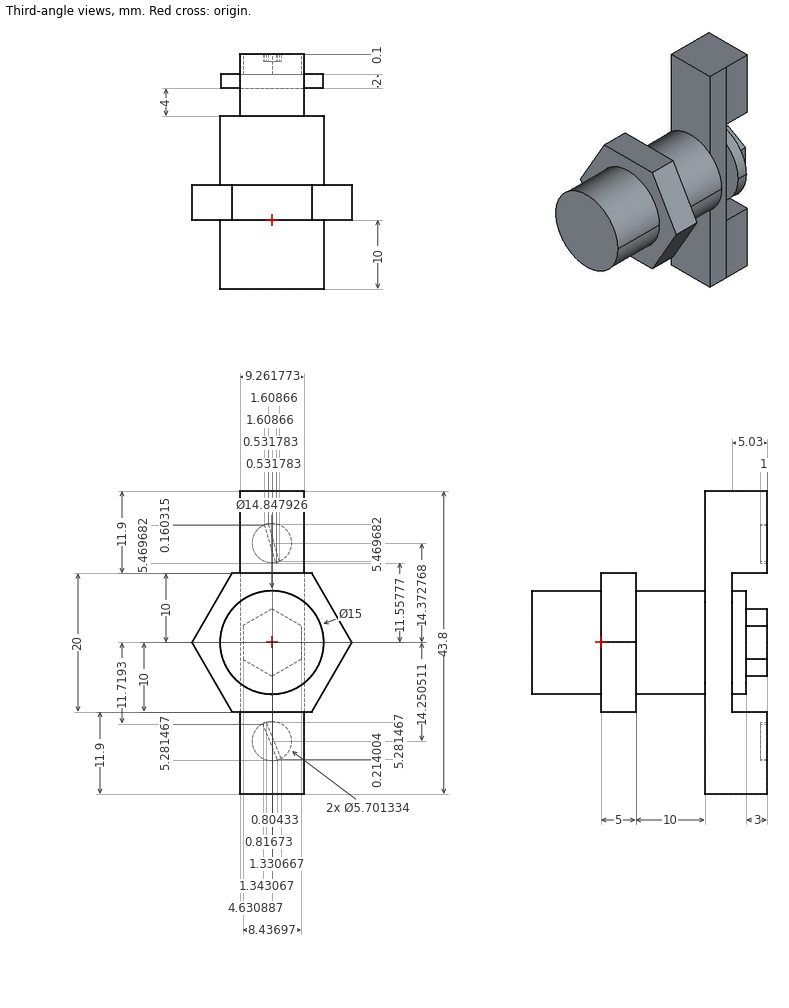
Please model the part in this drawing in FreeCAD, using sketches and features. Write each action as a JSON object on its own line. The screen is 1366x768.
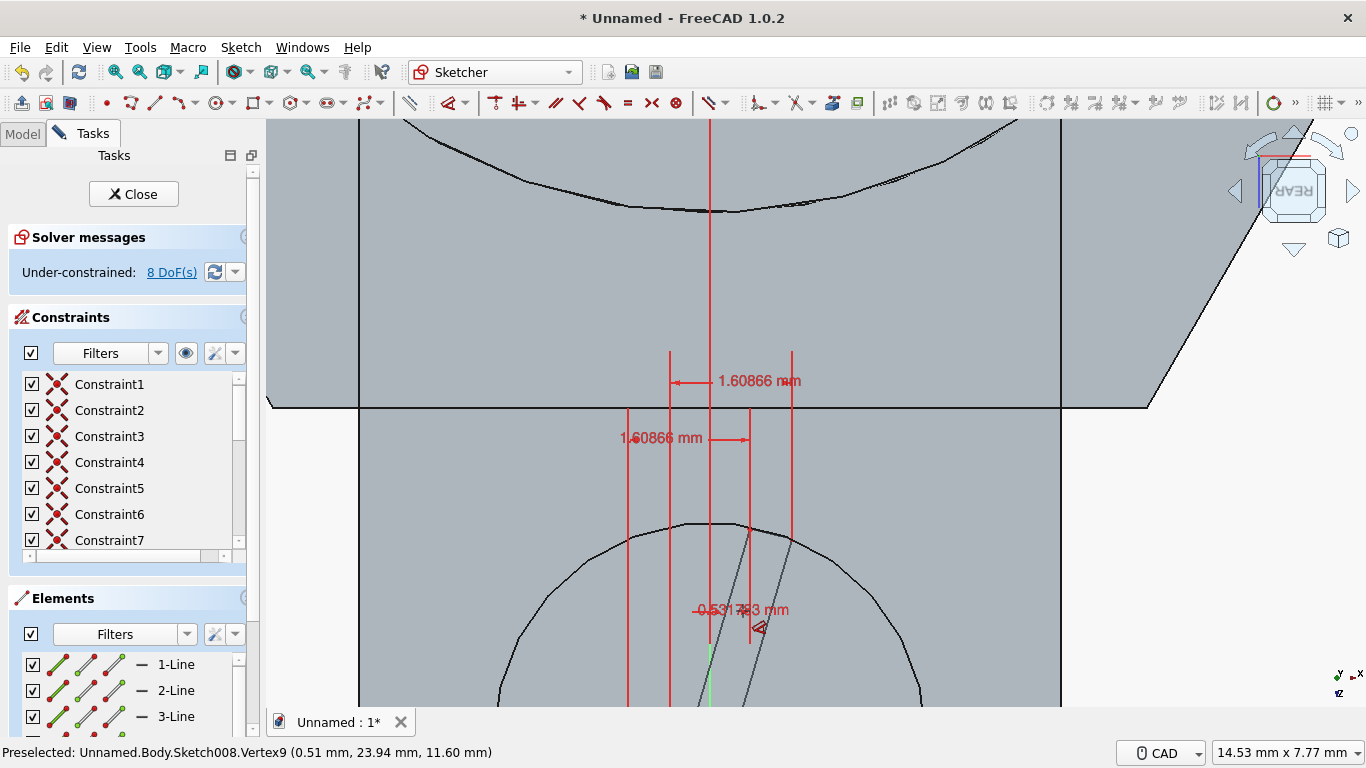
{"action": "scroll", "coordinate": [753, 531], "scroll_direction": "down", "scroll_amount": 10}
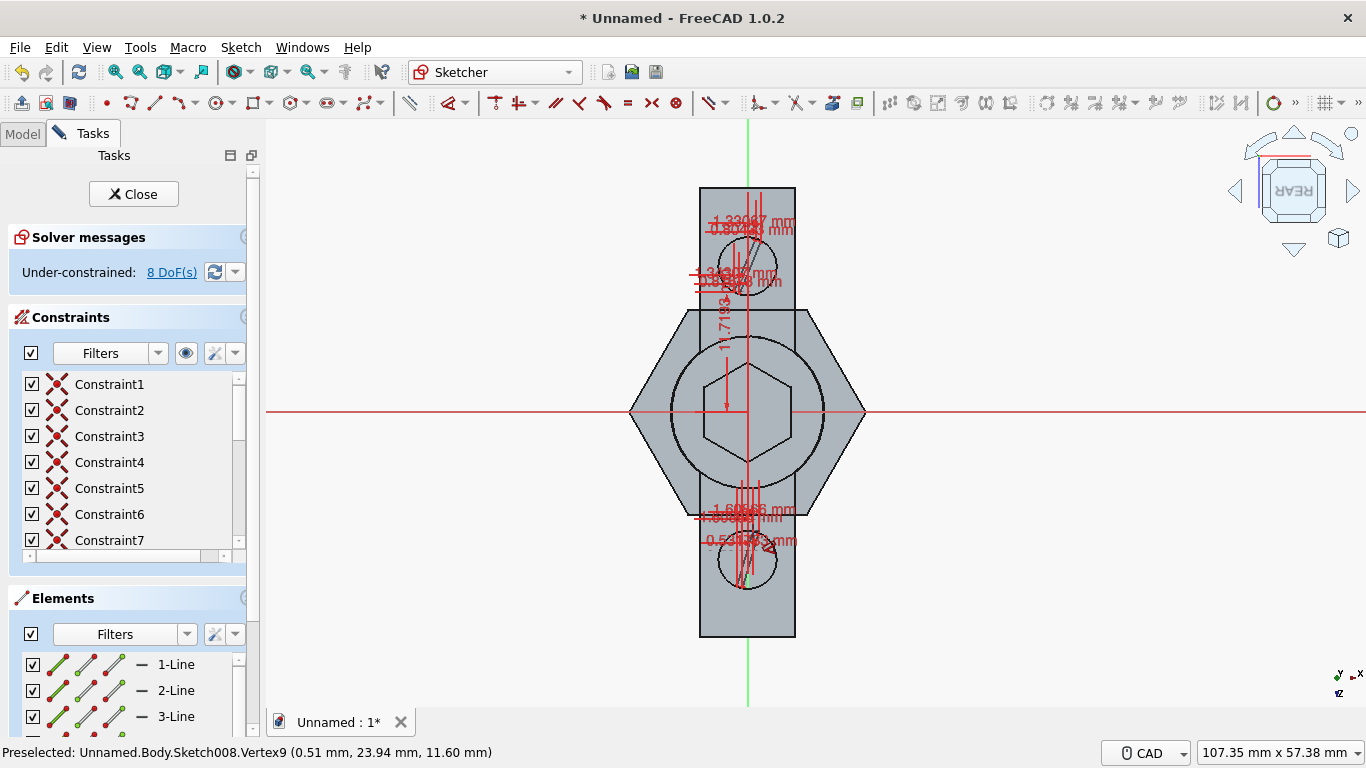
{"action": "scroll", "coordinate": [753, 531], "scroll_direction": "up", "scroll_amount": 4}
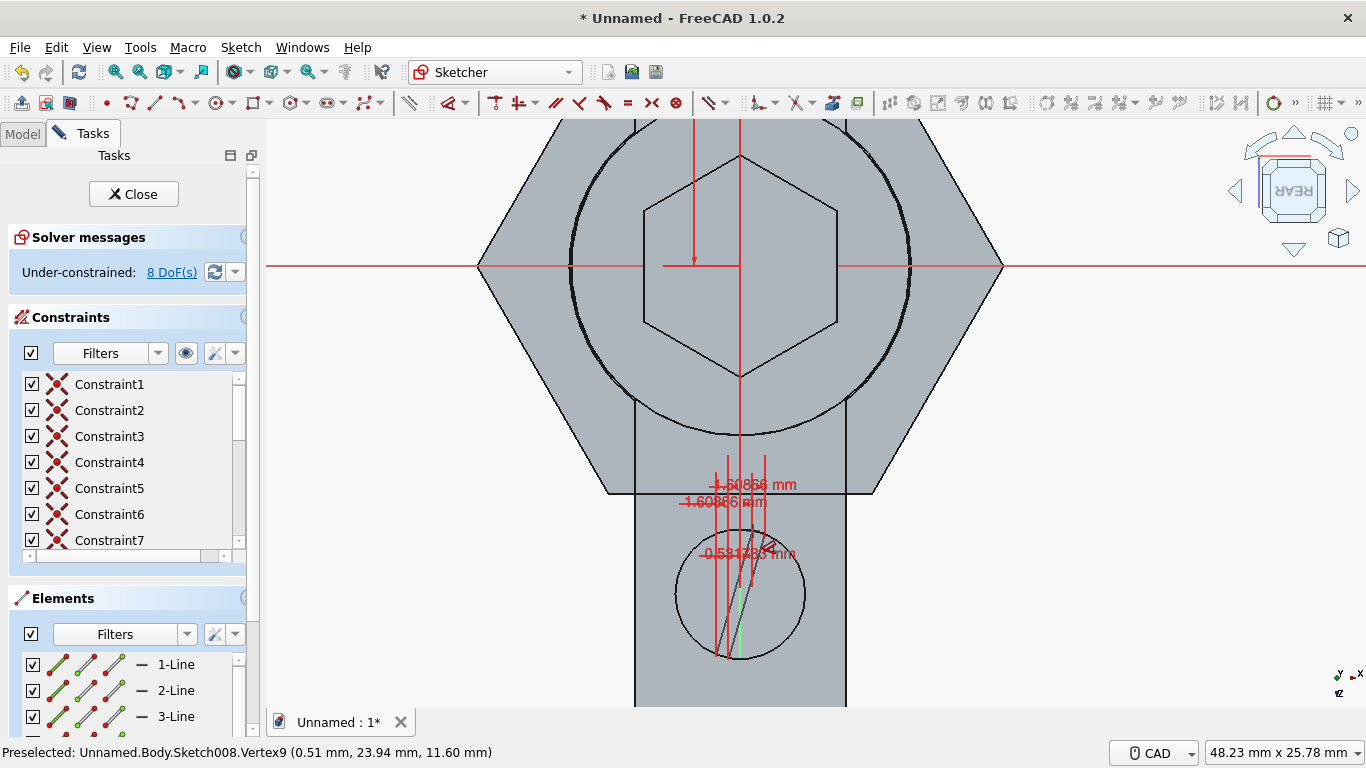
{"action": "left_click", "coordinate": [752, 531]}
{"action": "left_click", "coordinate": [786, 399]}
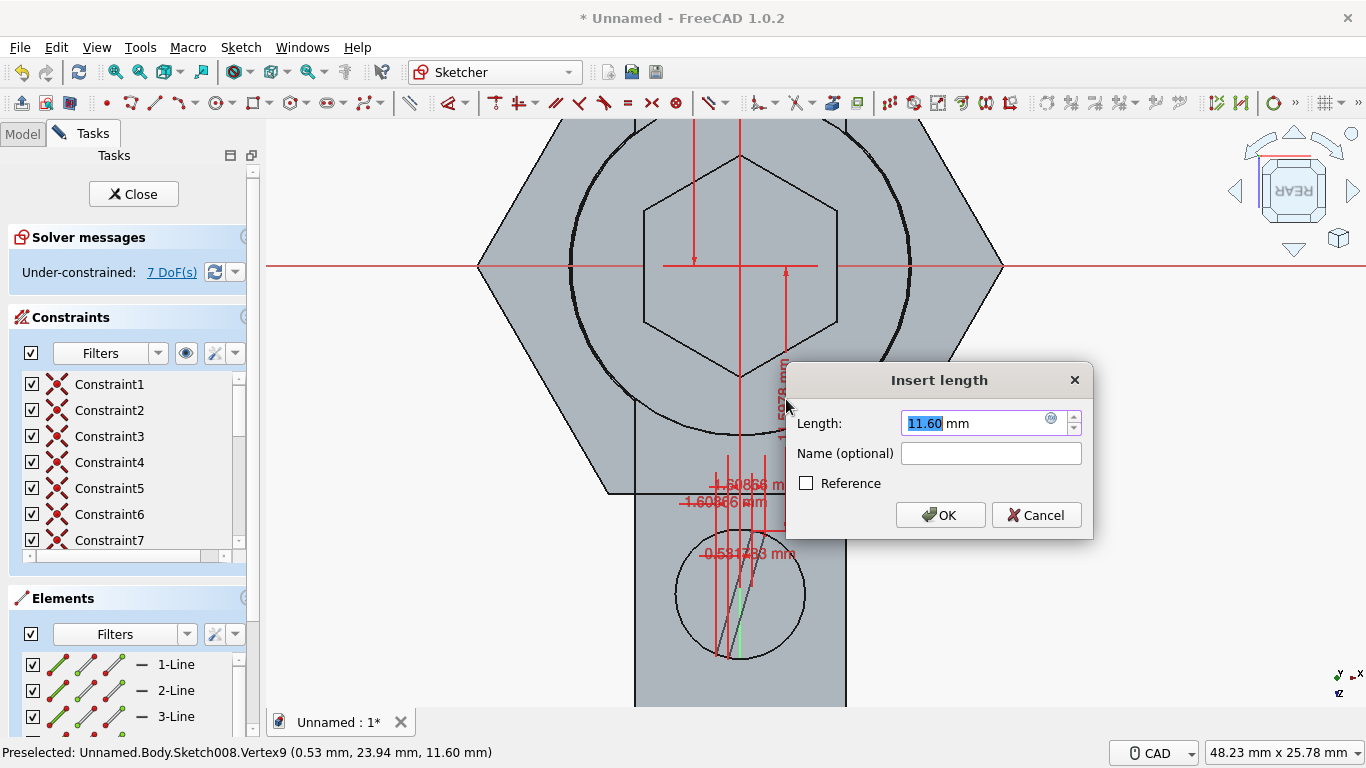
{"action": "type", "text": "11.55777"}
{"action": "key", "text": "Return"}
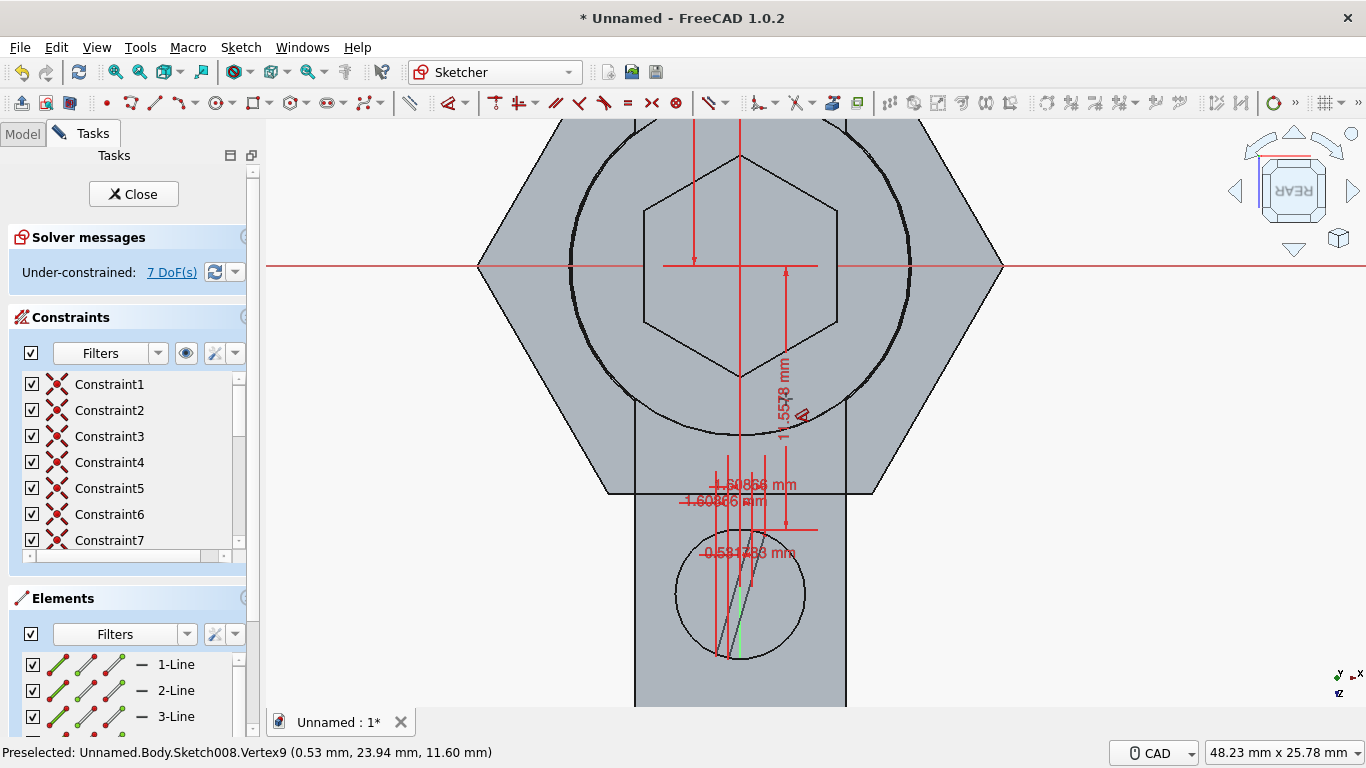
{"action": "scroll", "coordinate": [728, 659], "scroll_direction": "up", "scroll_amount": 6}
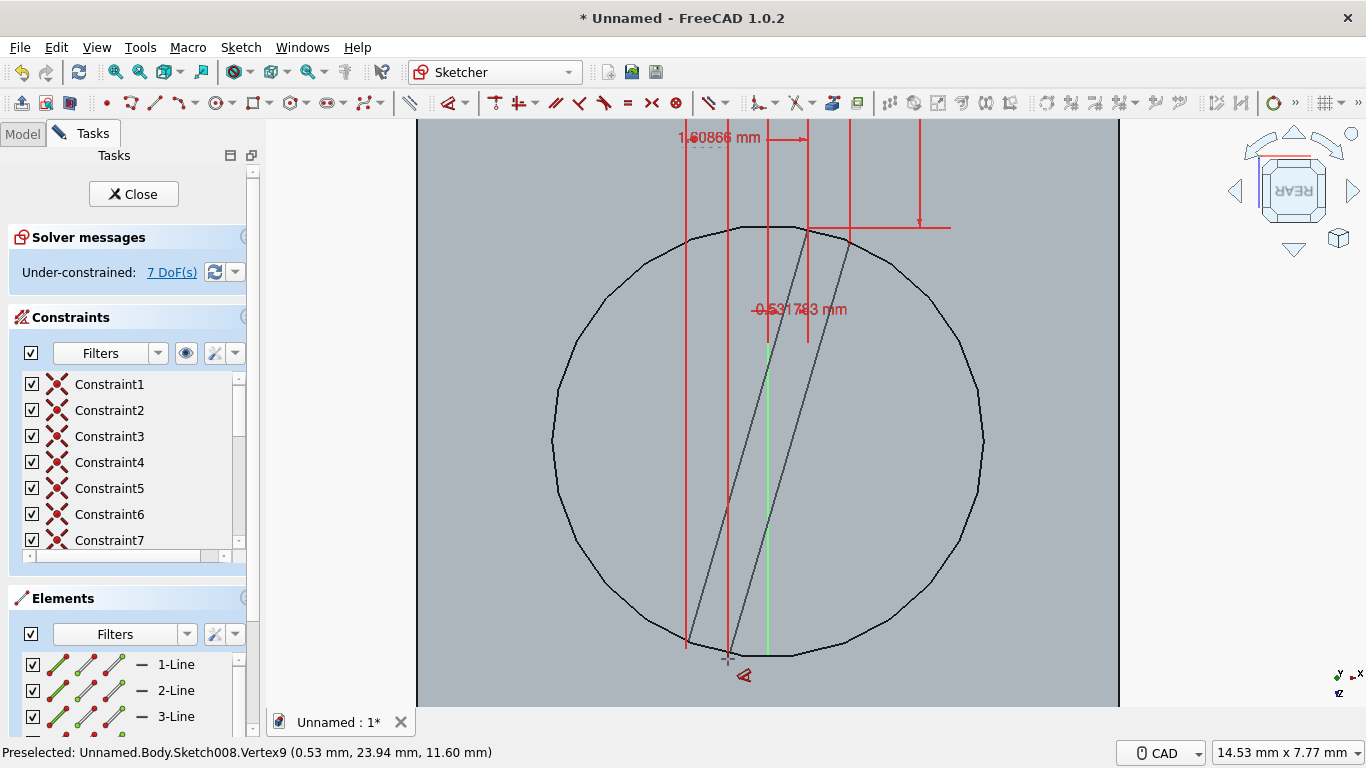
{"action": "left_click", "coordinate": [728, 658]}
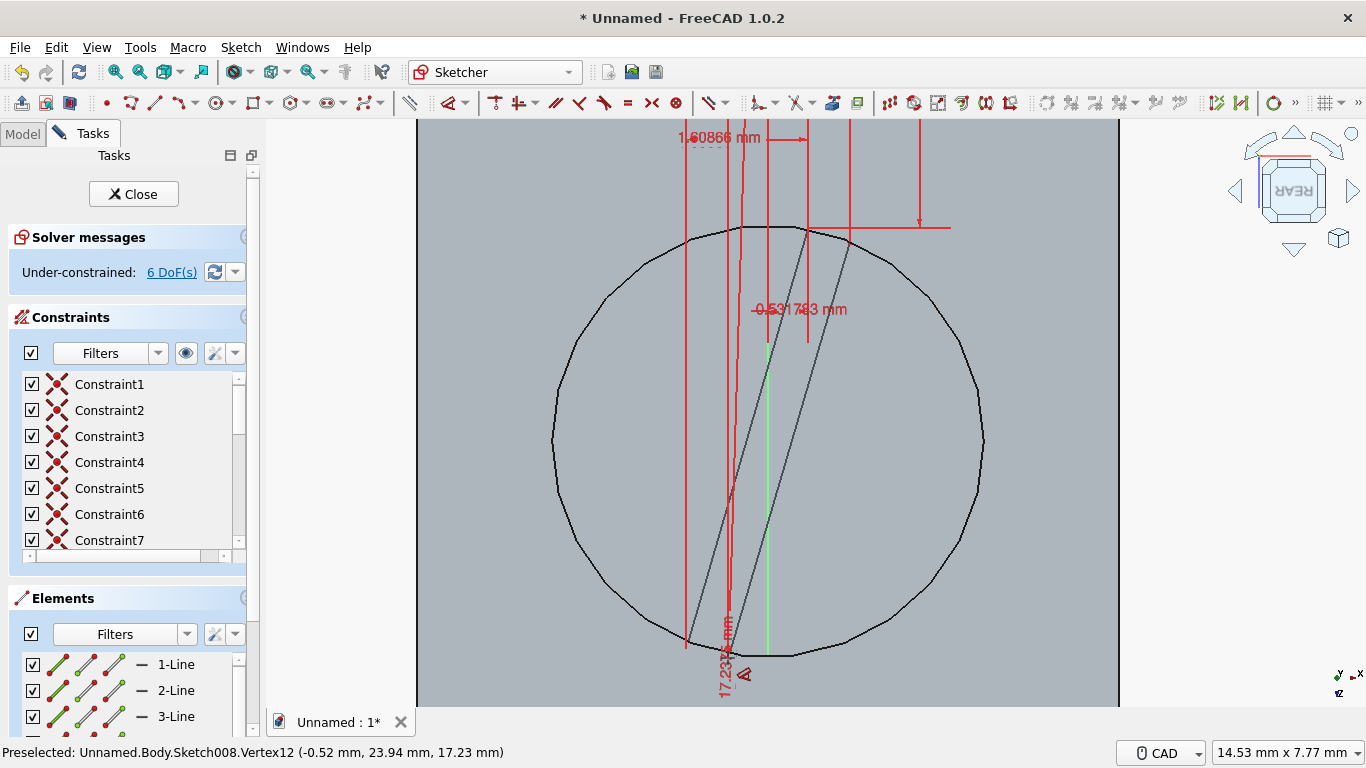
{"action": "key", "text": "Escape"}
{"action": "key", "text": "Escape"}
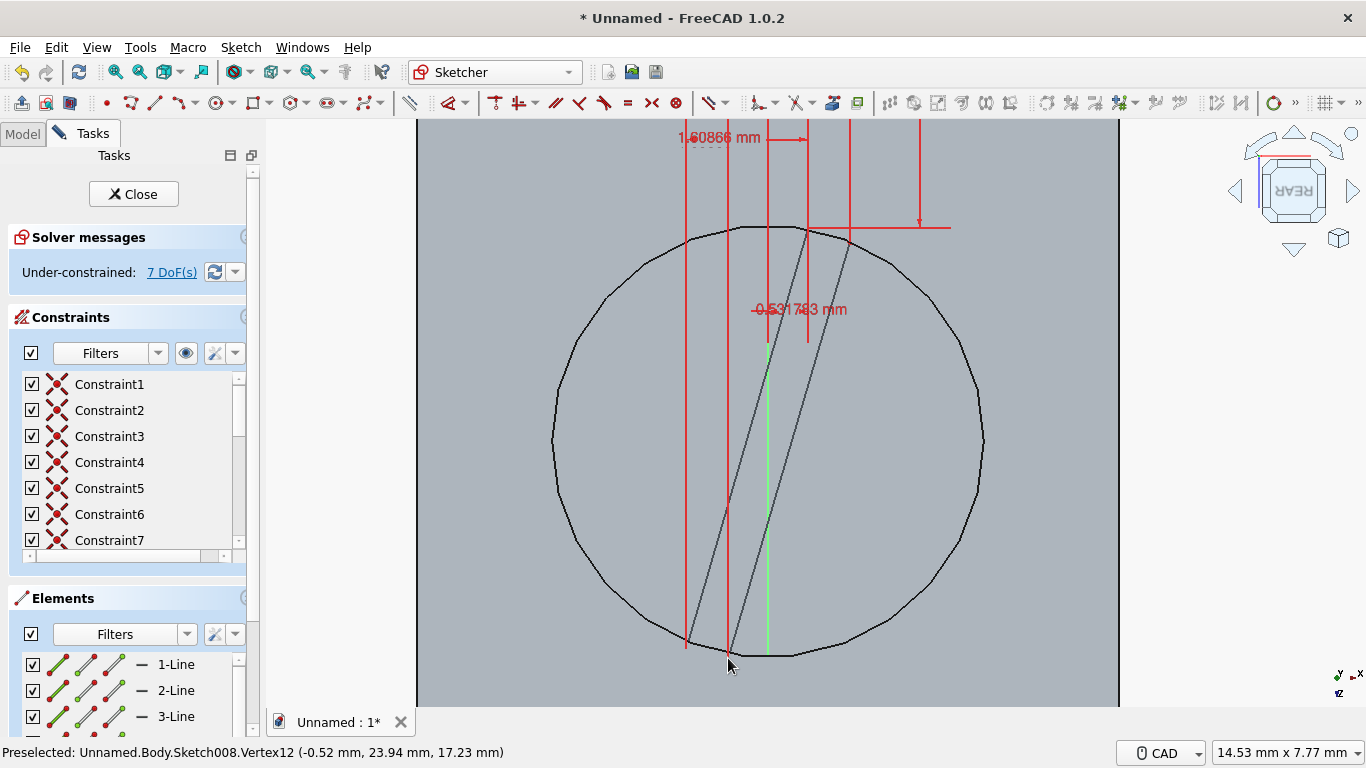
{"action": "left_click", "coordinate": [728, 658]}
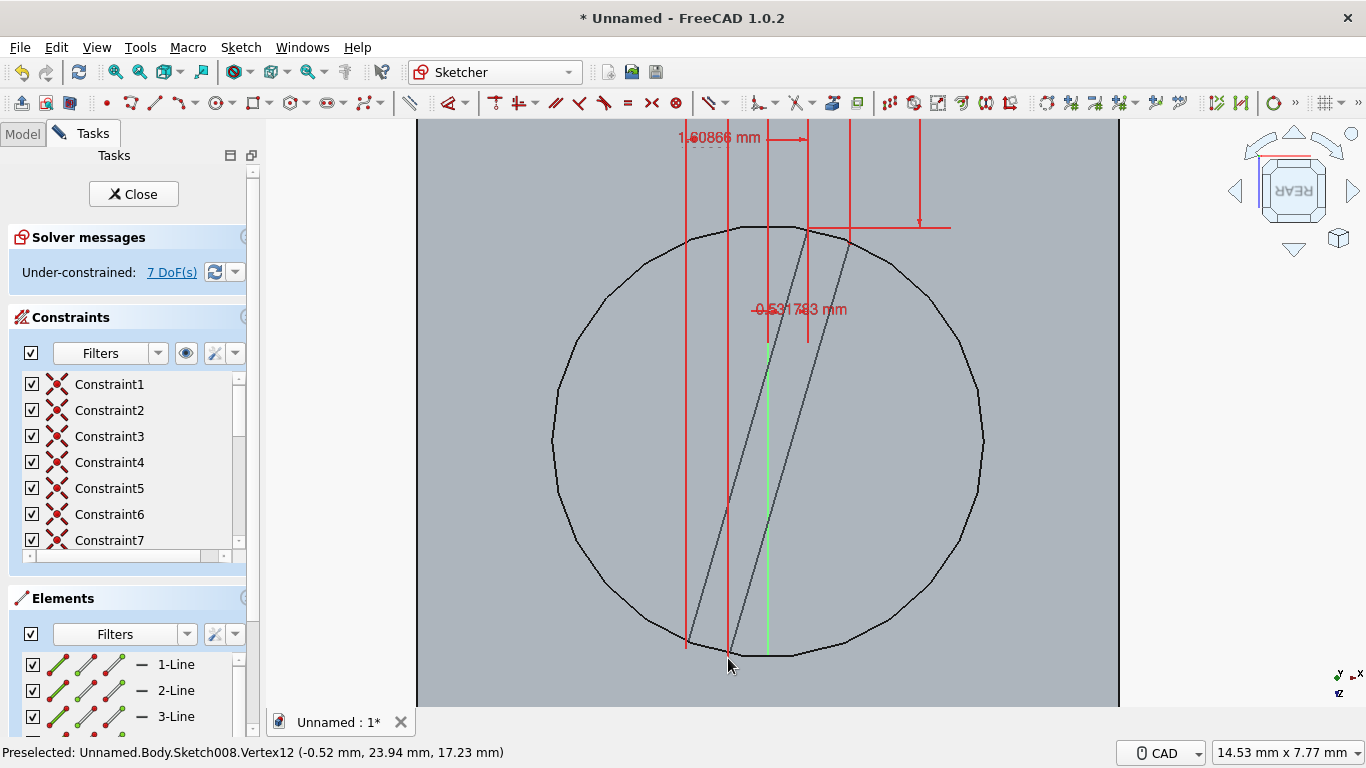
{"action": "left_click", "coordinate": [468, 104]}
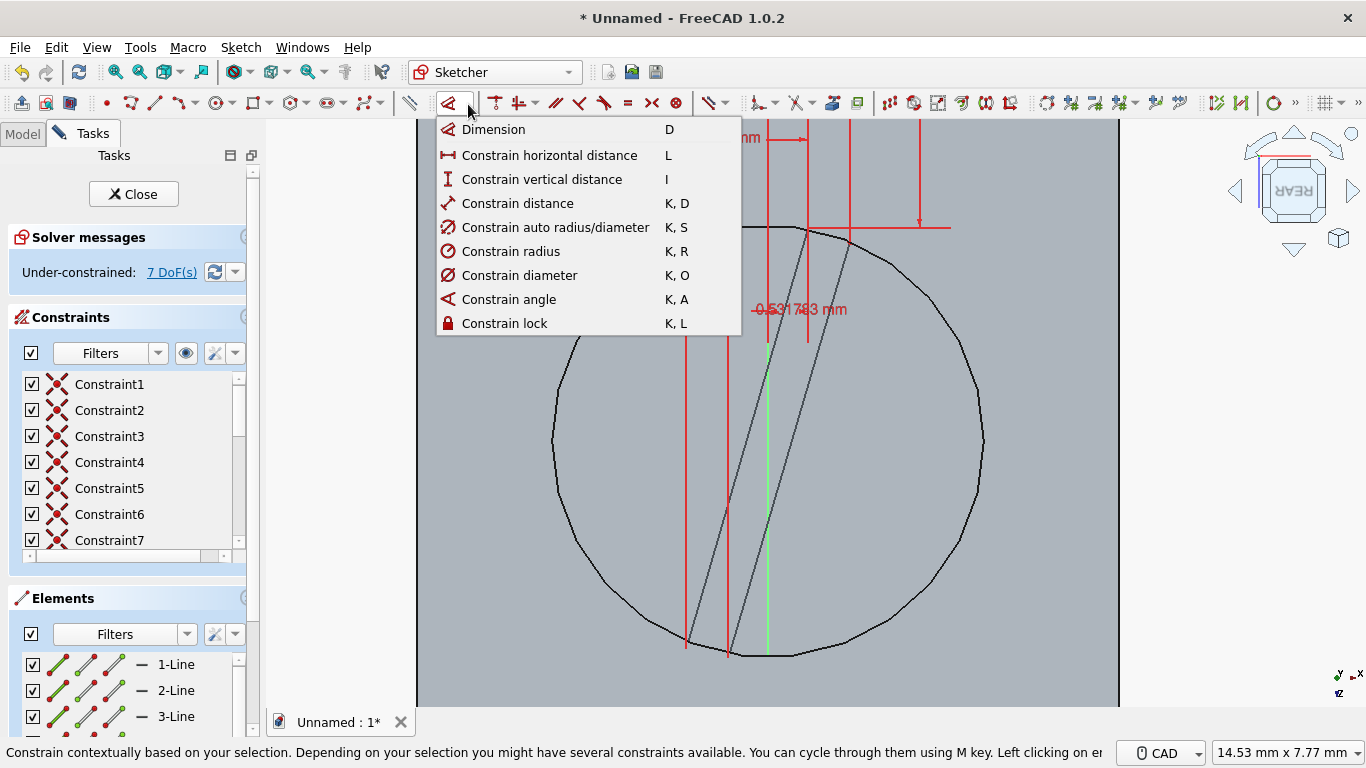
{"action": "left_click", "coordinate": [589, 155]}